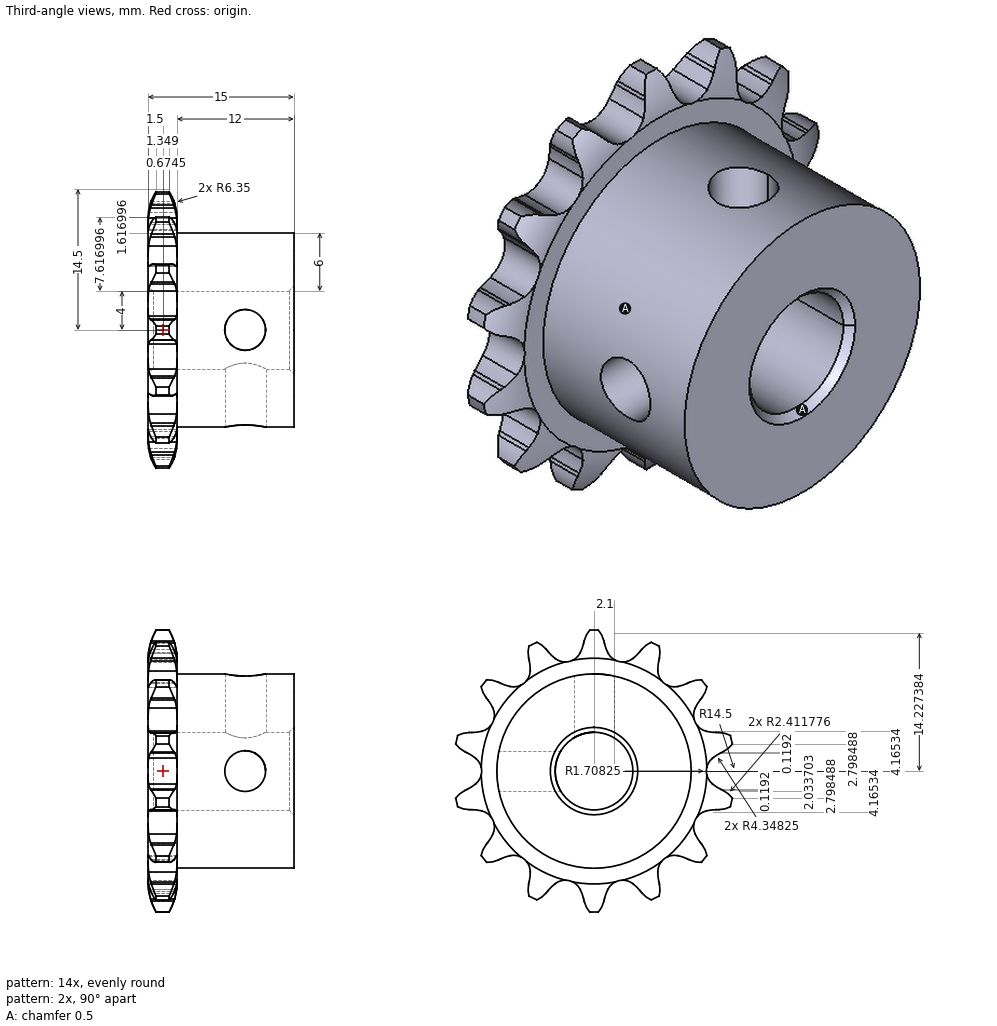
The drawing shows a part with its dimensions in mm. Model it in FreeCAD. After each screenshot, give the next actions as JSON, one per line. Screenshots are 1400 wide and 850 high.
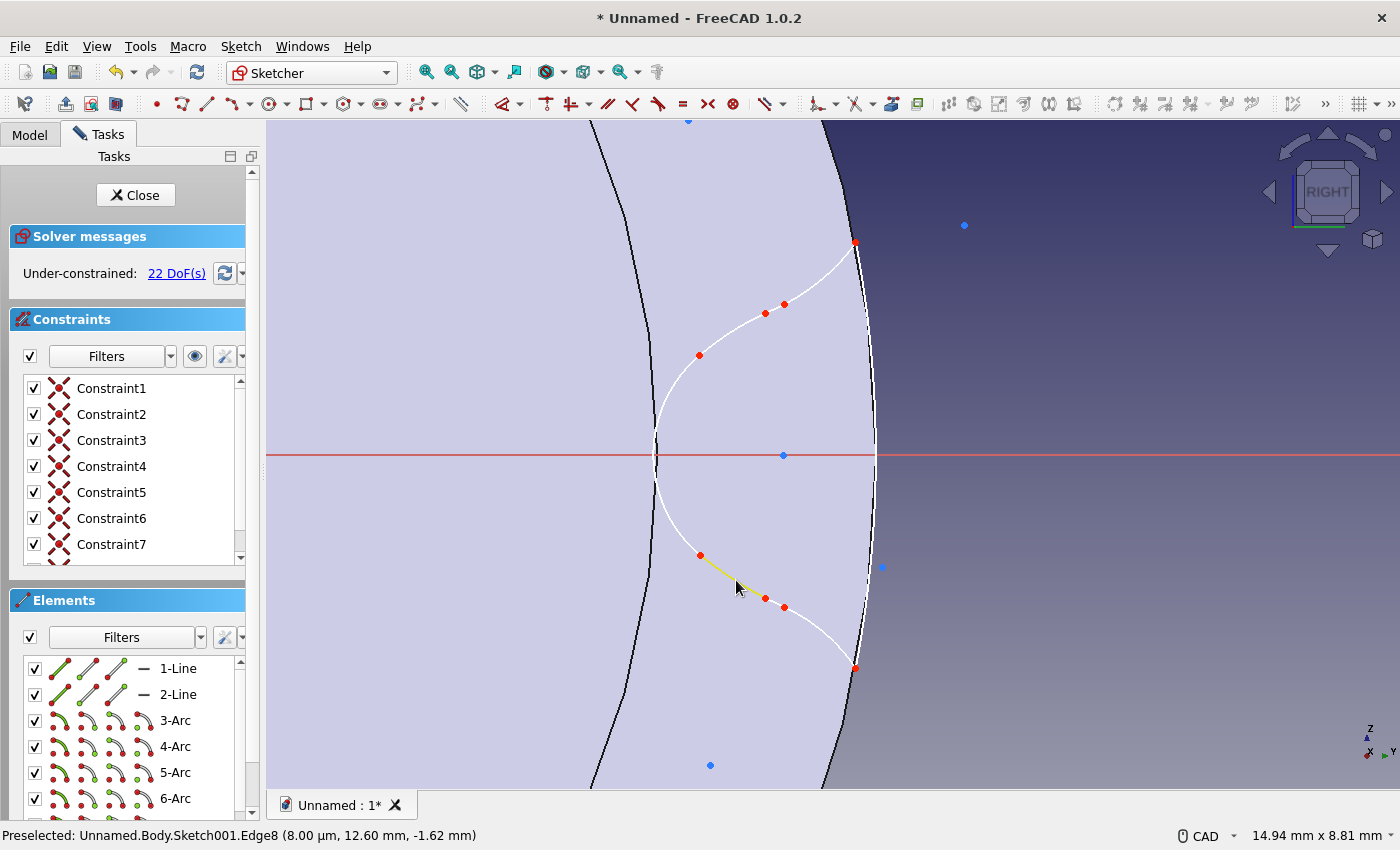
{"action": "scroll", "coordinate": [771, 601], "scroll_direction": "up", "scroll_amount": 4}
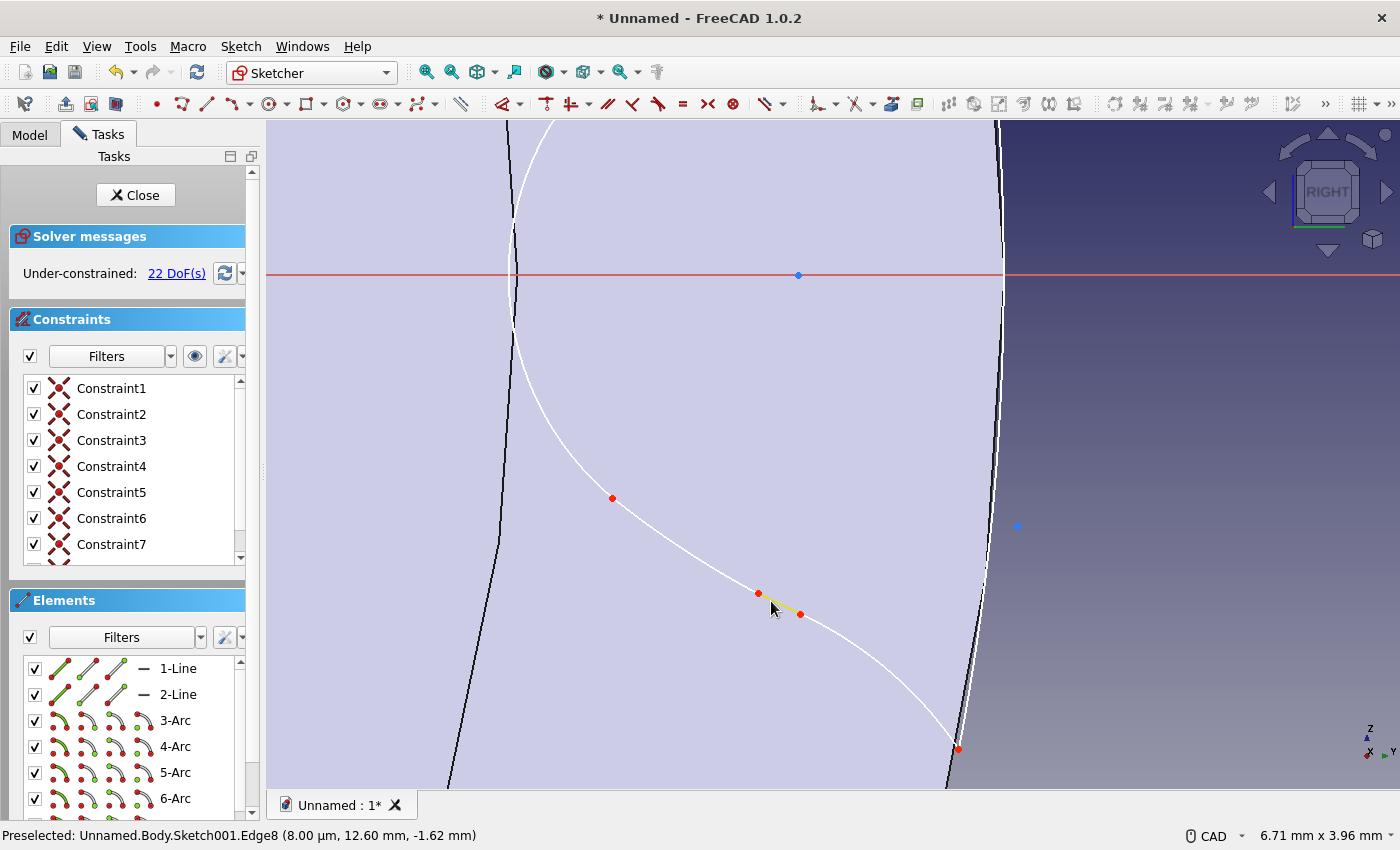
{"action": "left_click", "coordinate": [771, 600]}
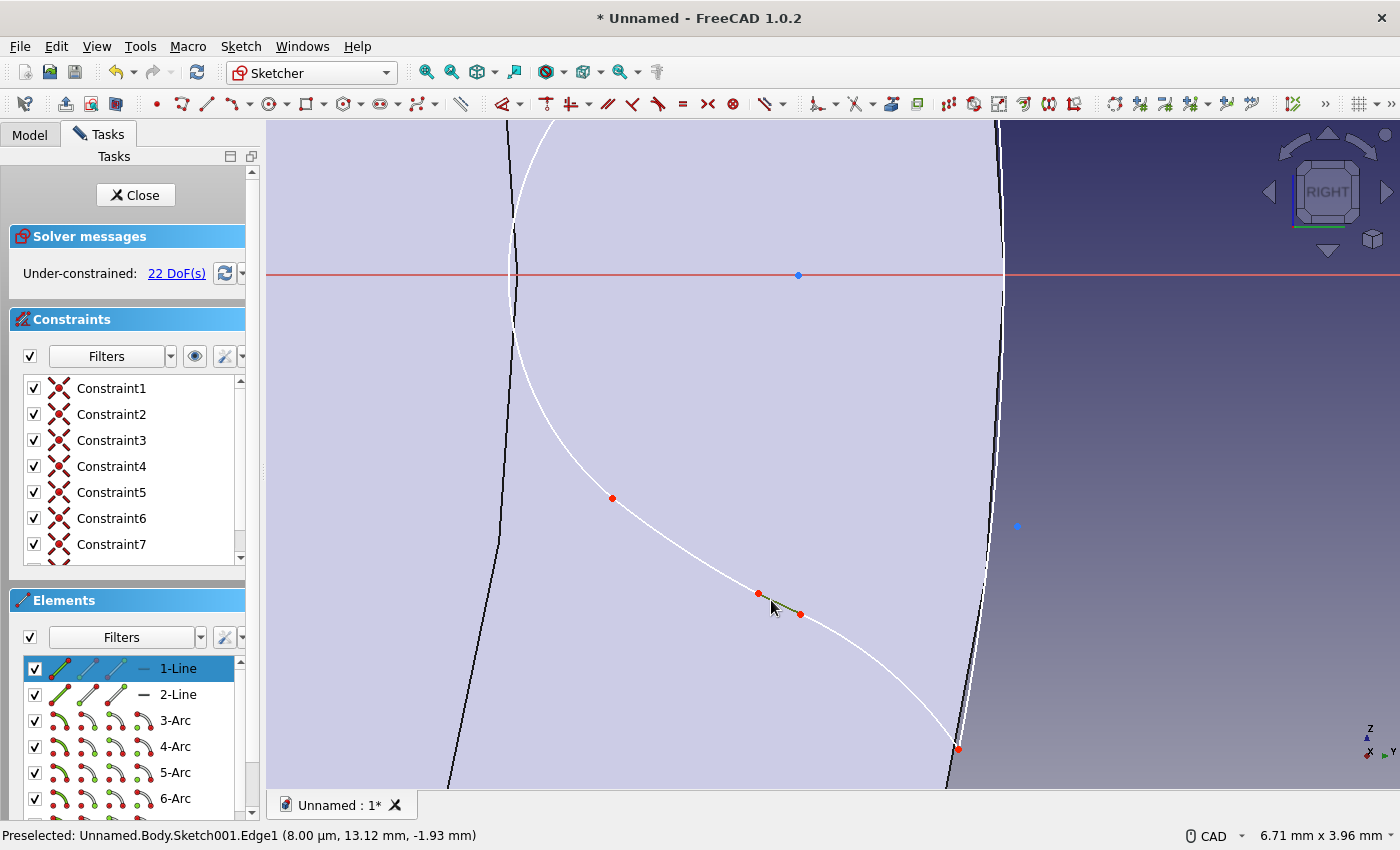
{"action": "left_click", "coordinate": [919, 700]}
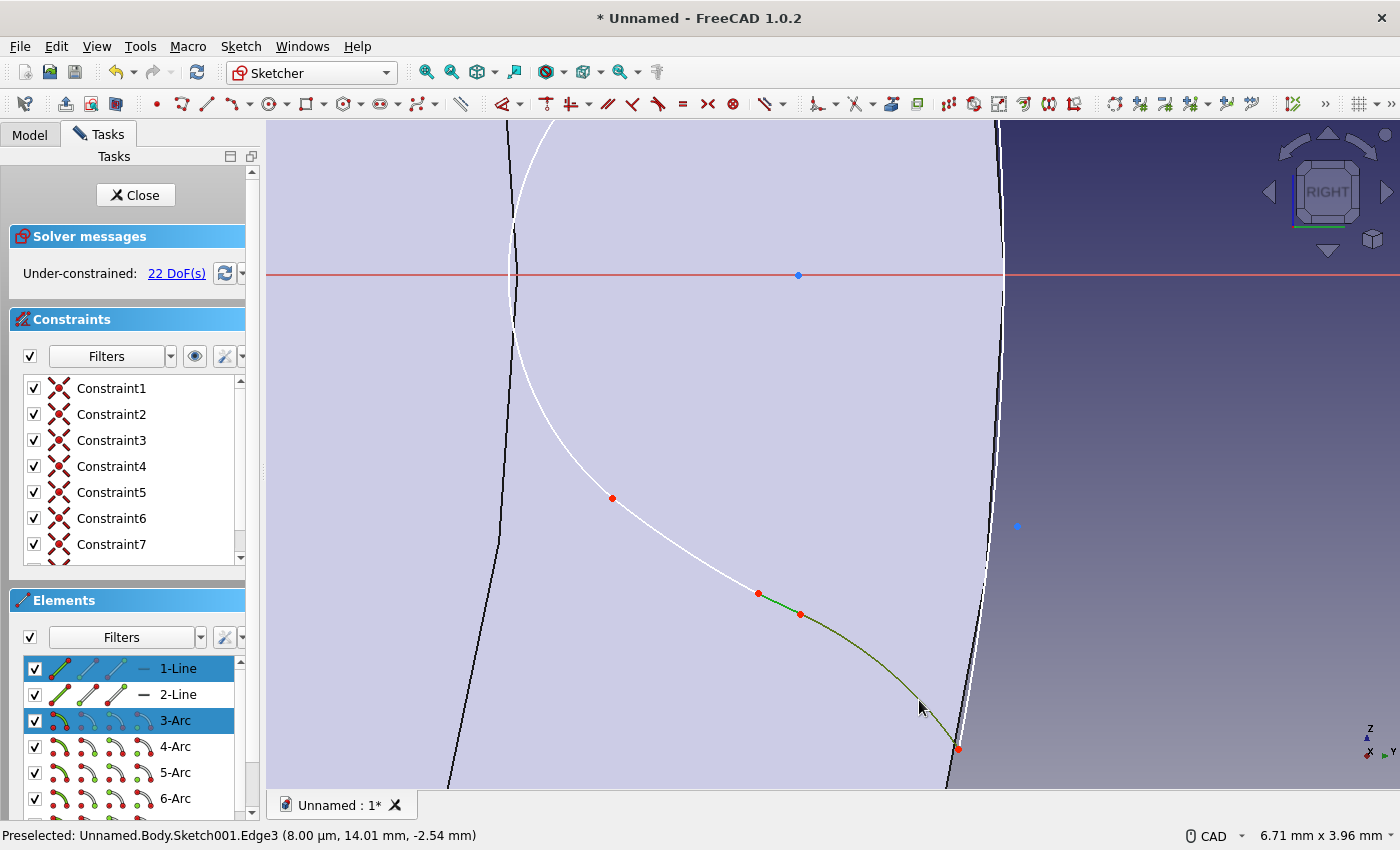
{"action": "left_click", "coordinate": [658, 104]}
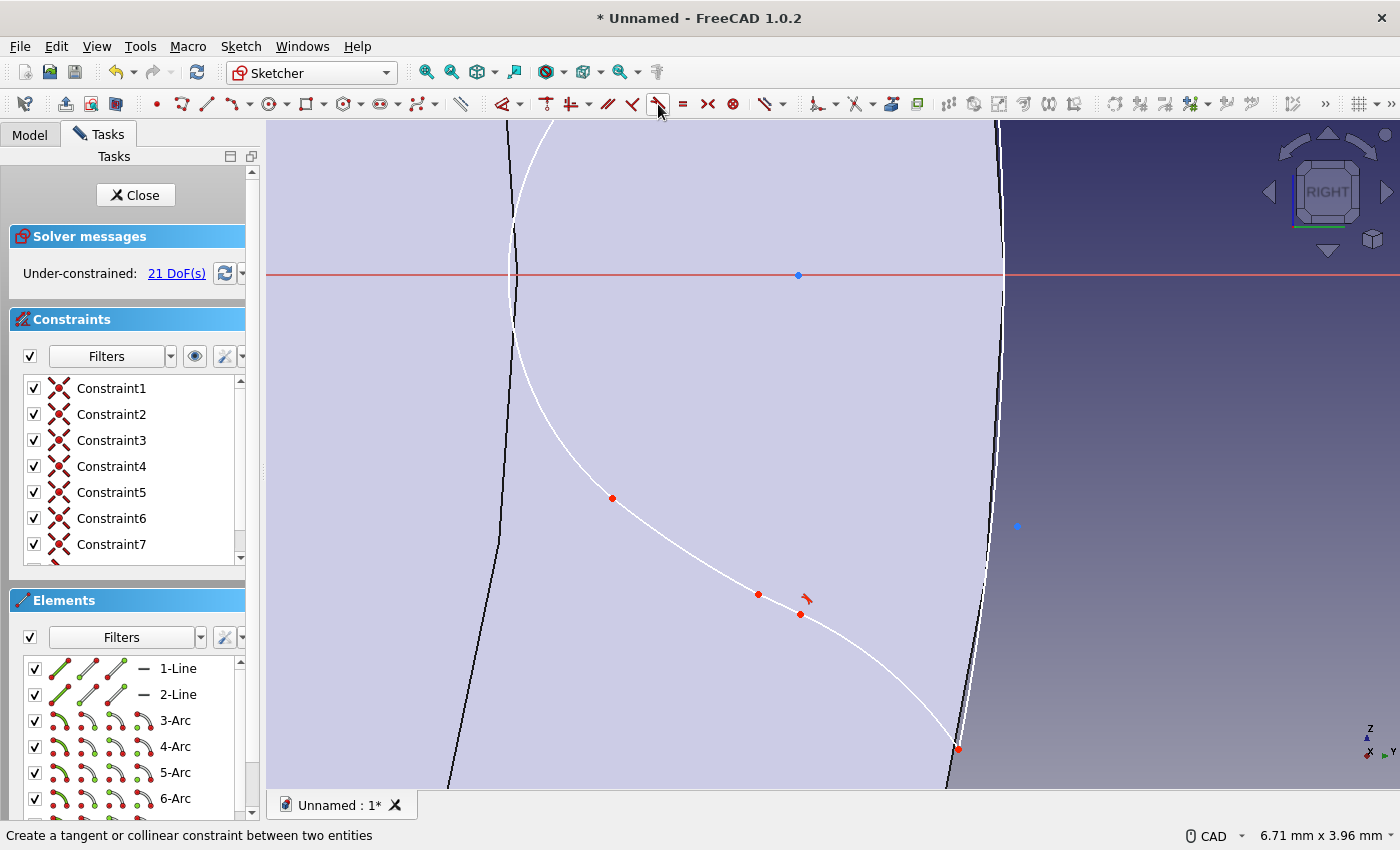
{"action": "left_click", "coordinate": [771, 600]}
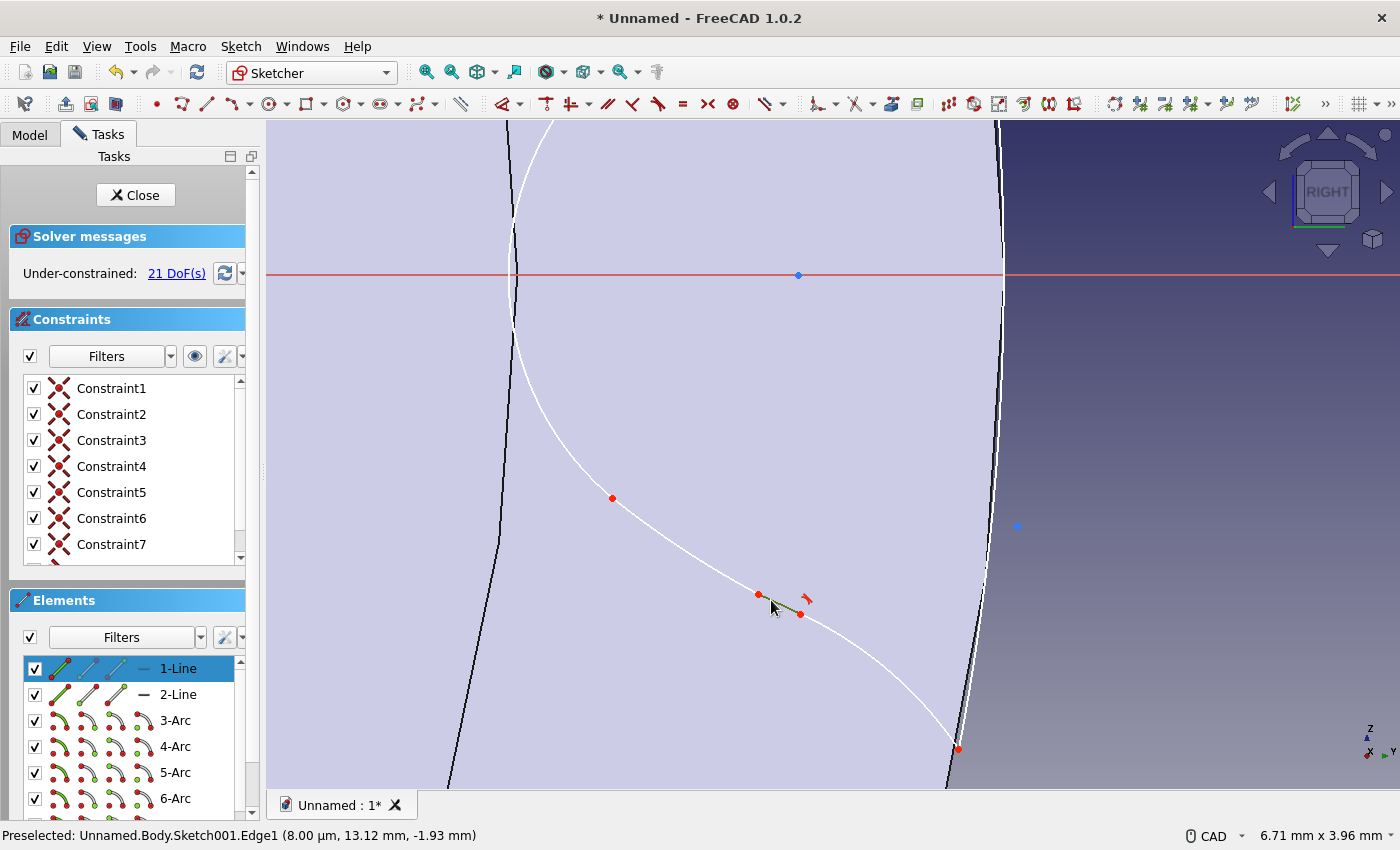
{"action": "left_click", "coordinate": [655, 530]}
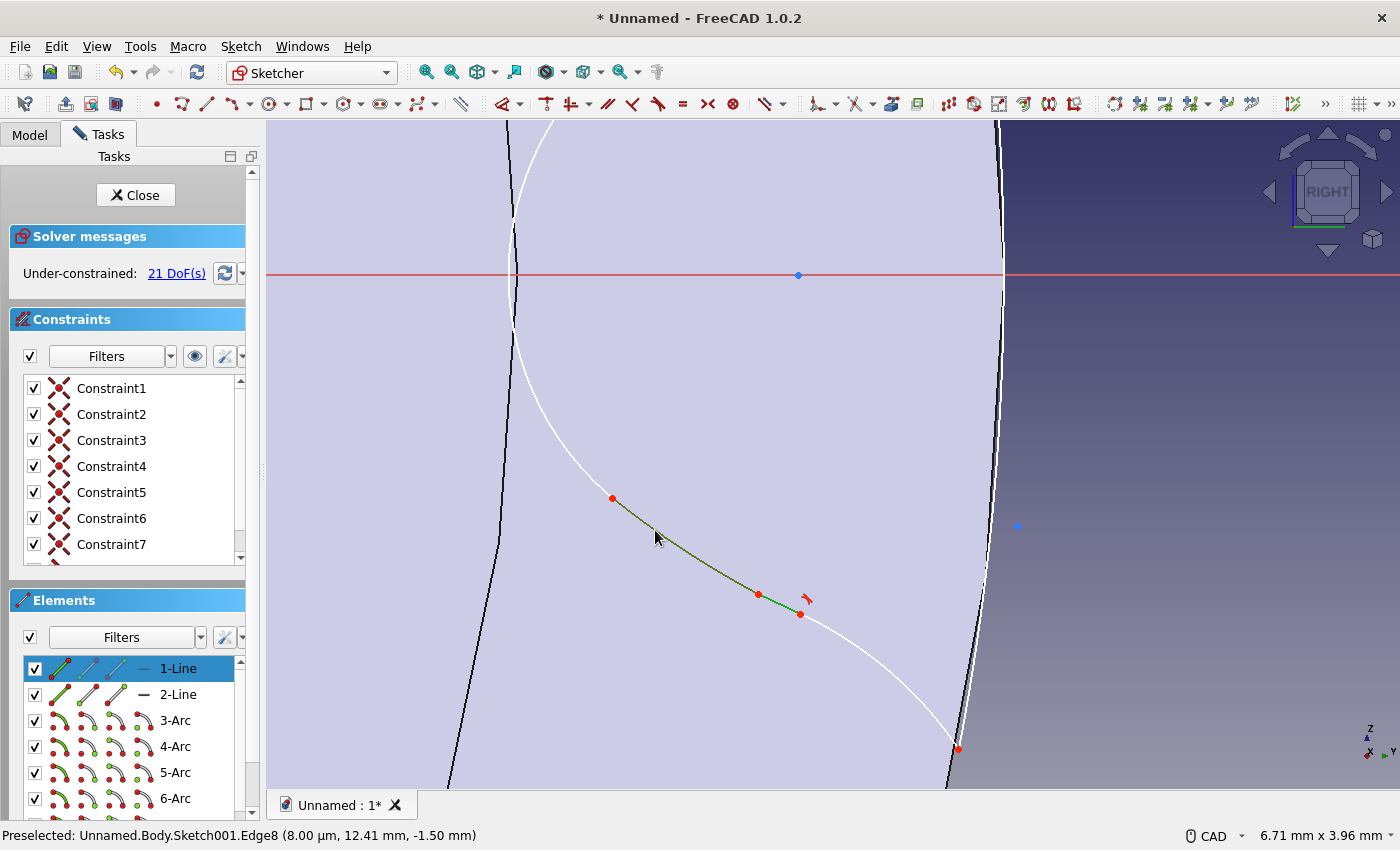
{"action": "left_click", "coordinate": [658, 104]}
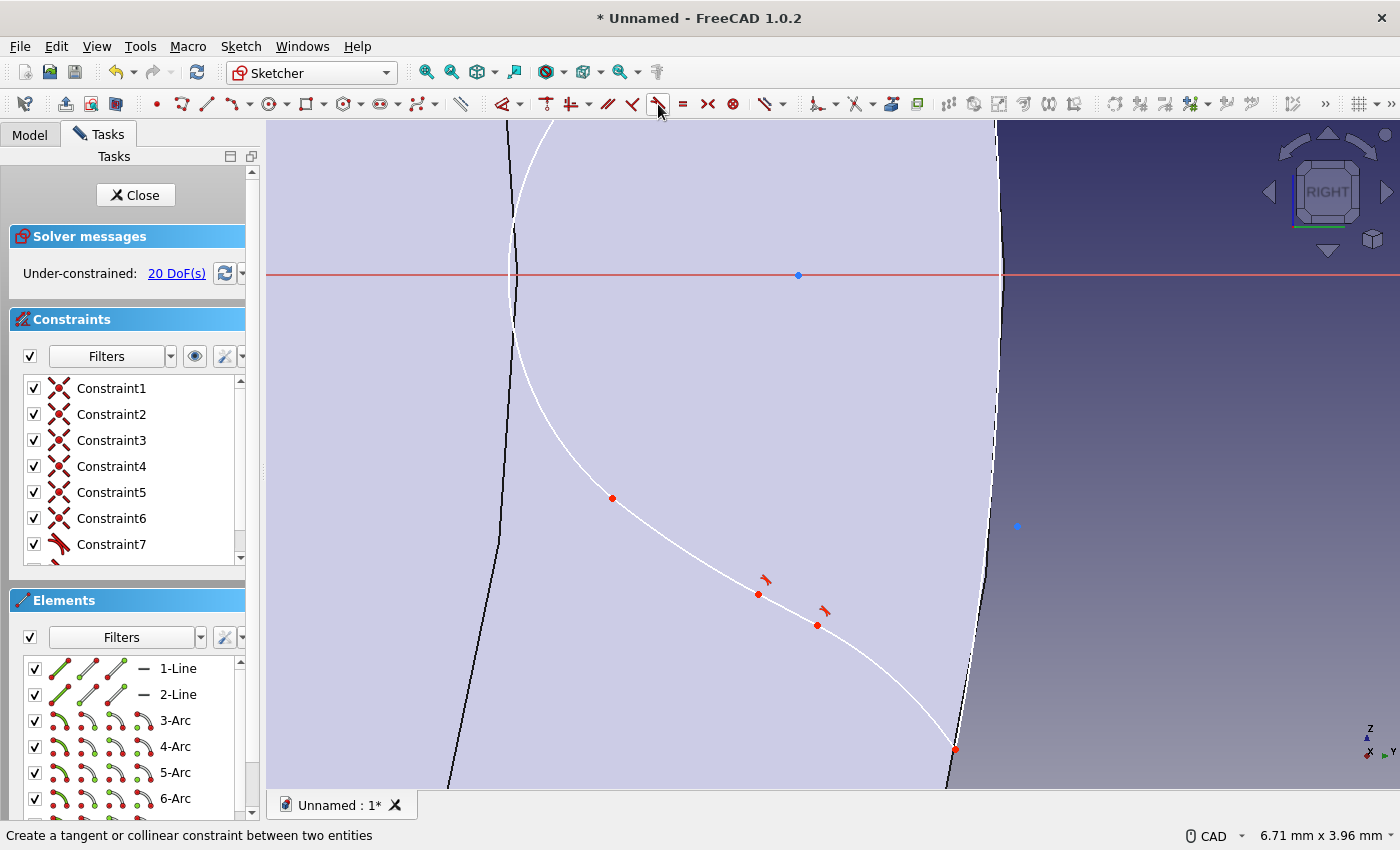
{"action": "scroll", "coordinate": [771, 601], "scroll_direction": "down", "scroll_amount": 4}